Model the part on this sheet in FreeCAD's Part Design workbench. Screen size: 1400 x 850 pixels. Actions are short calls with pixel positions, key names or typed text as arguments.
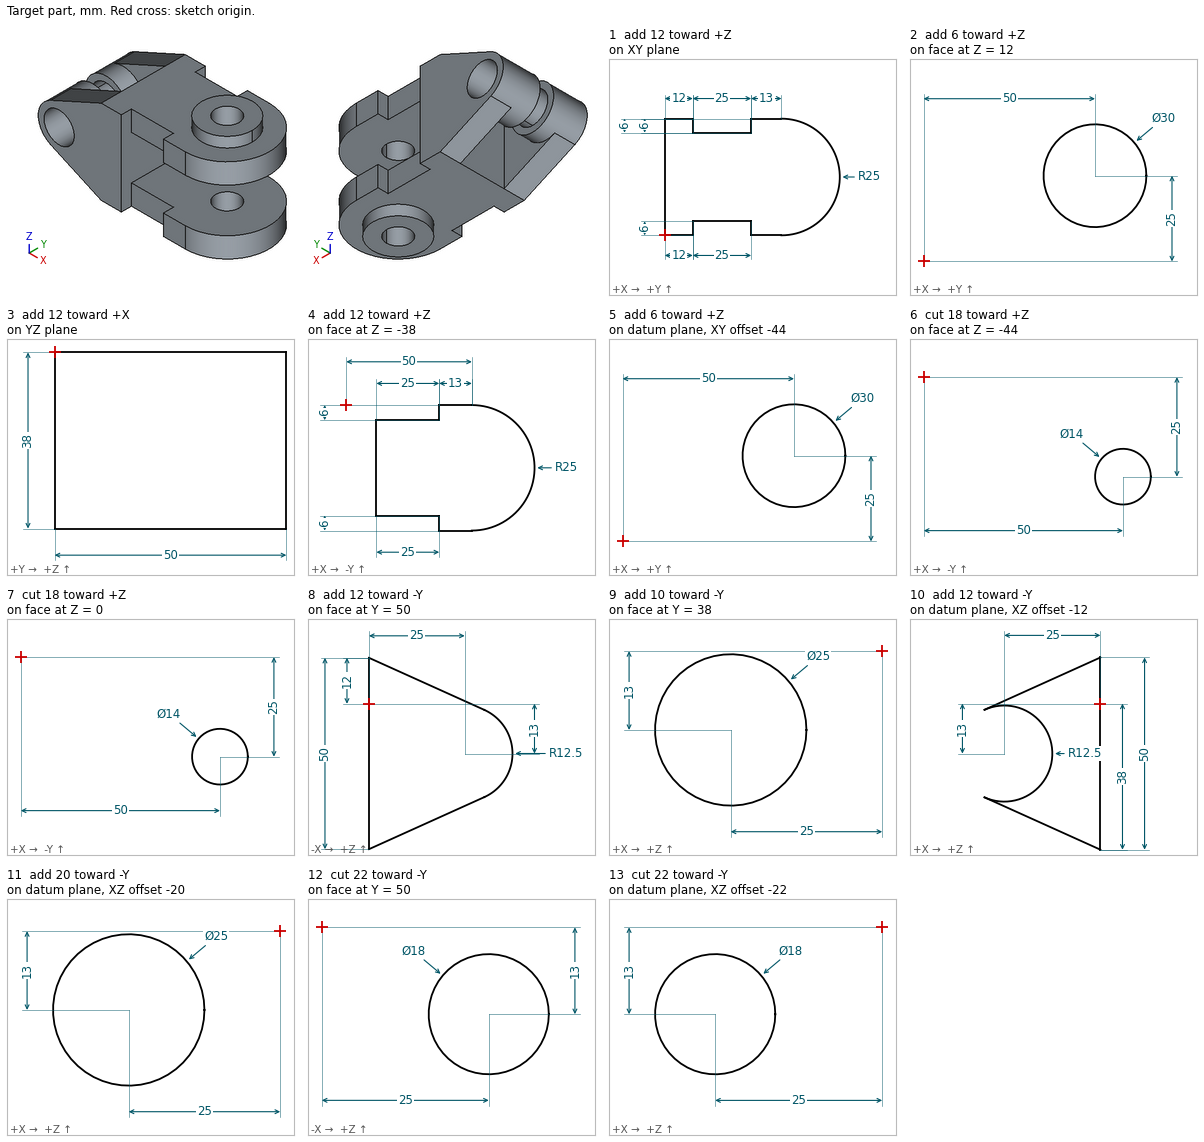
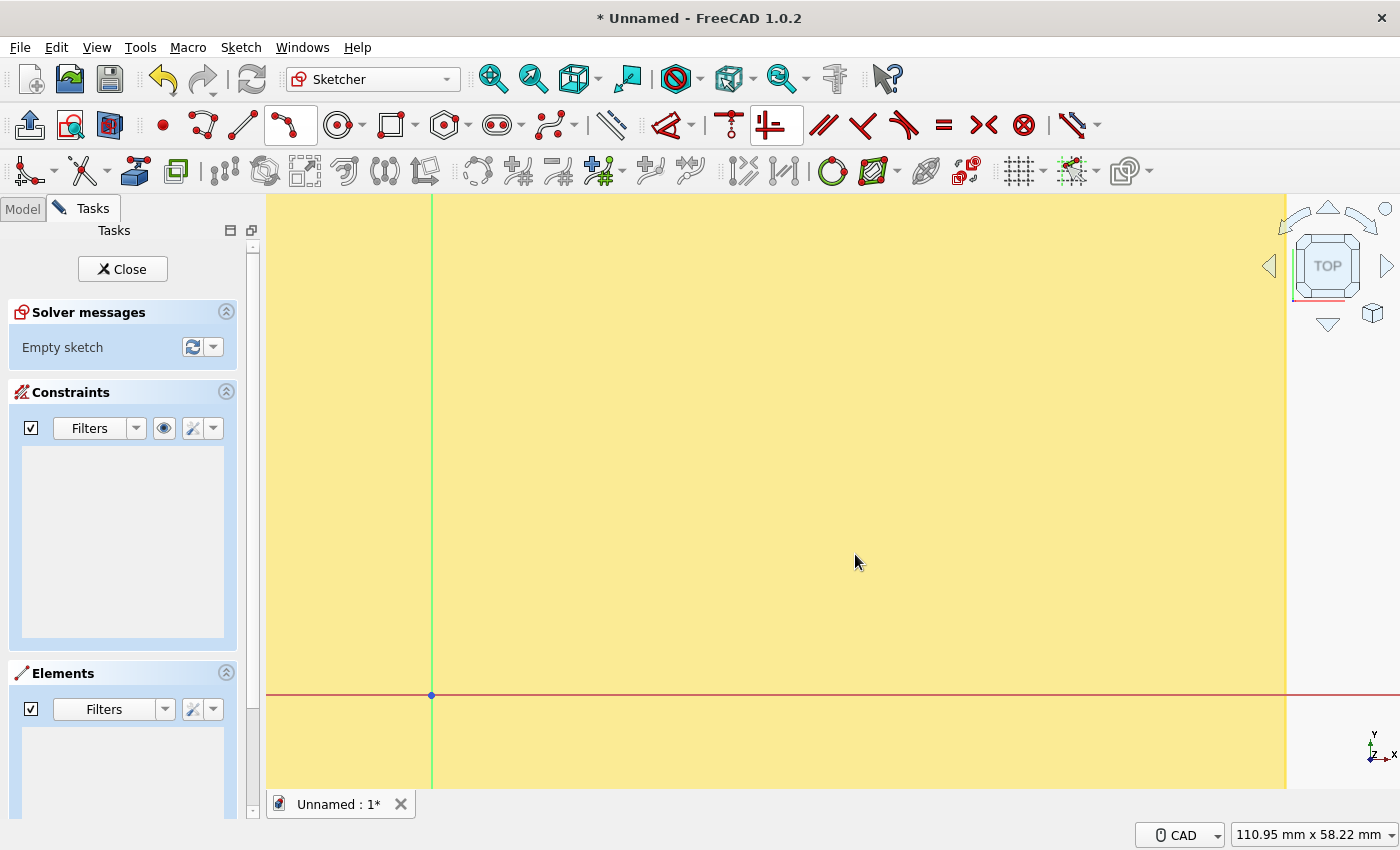
click(338, 126)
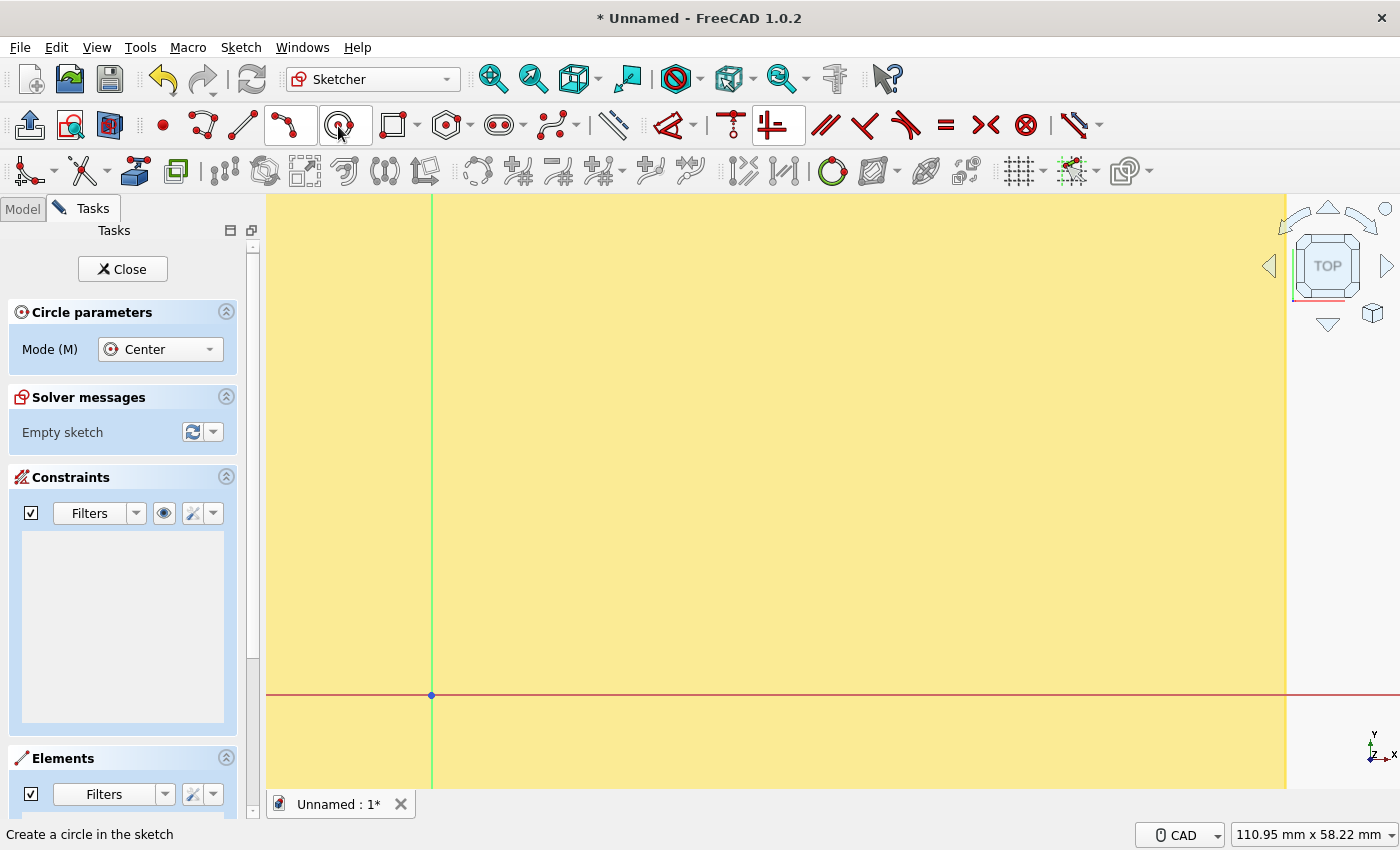
click(943, 440)
click(1051, 331)
key(Escape)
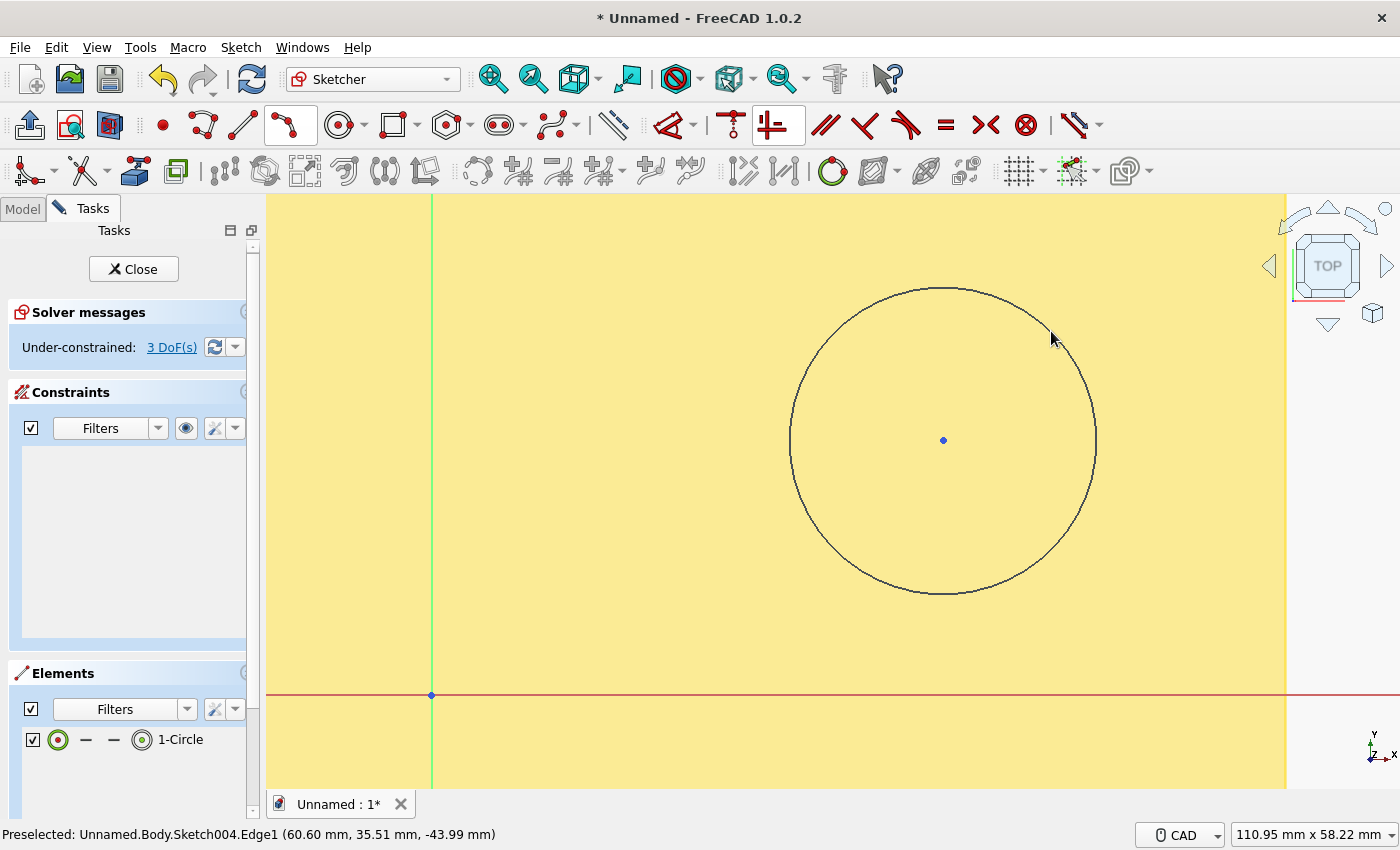
click(668, 126)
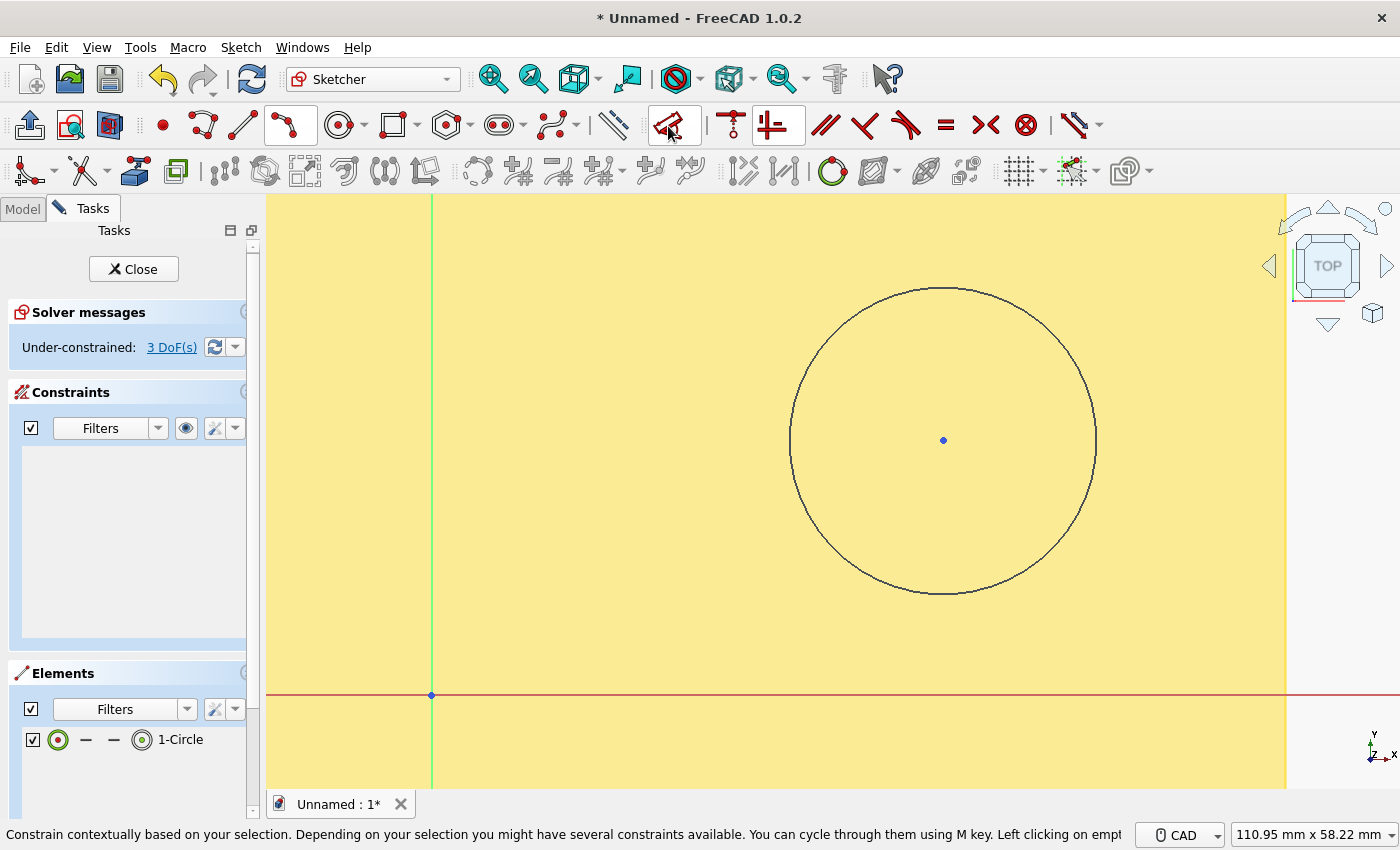
click(1051, 332)
click(1074, 309)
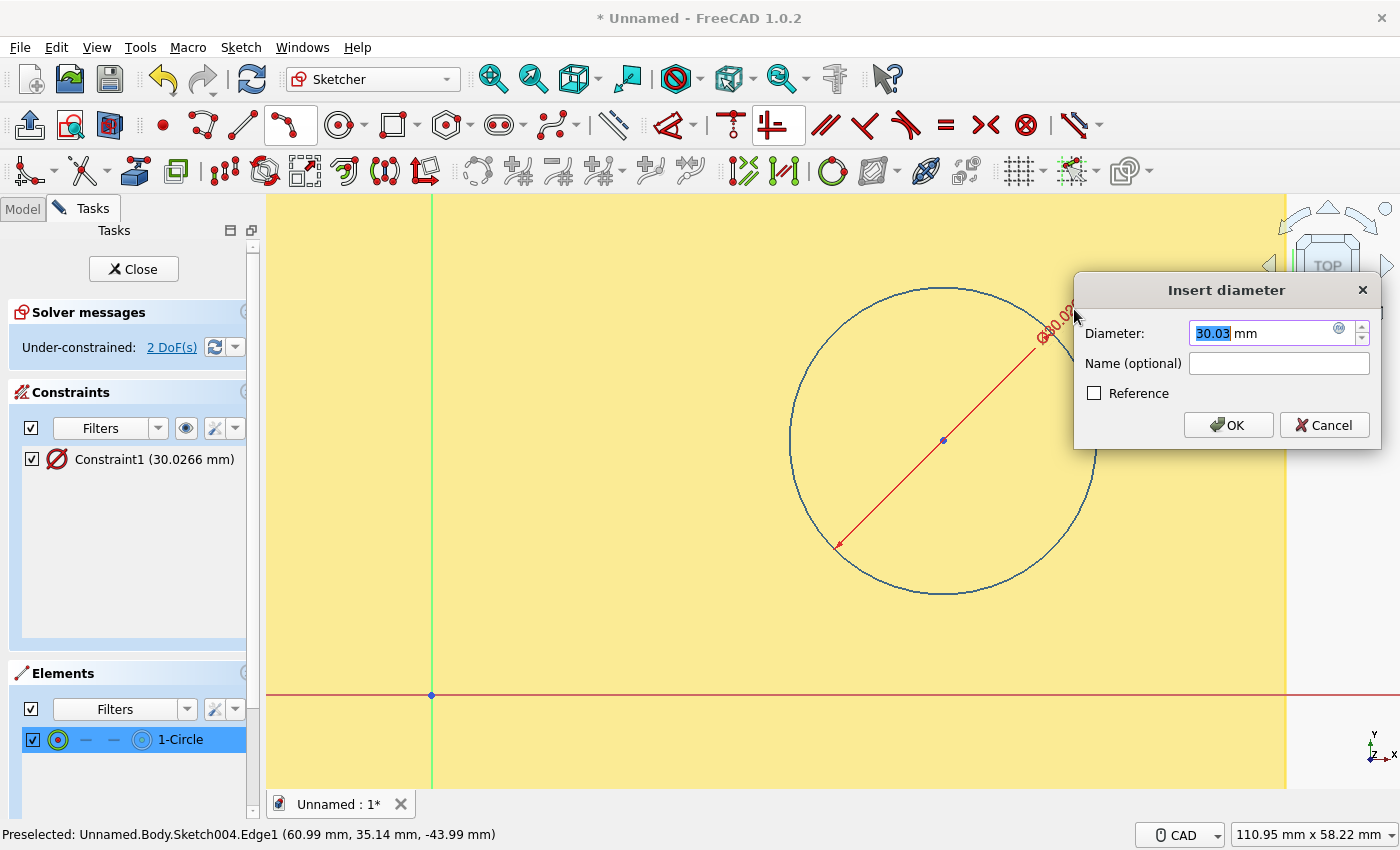
text(30)
key(Return)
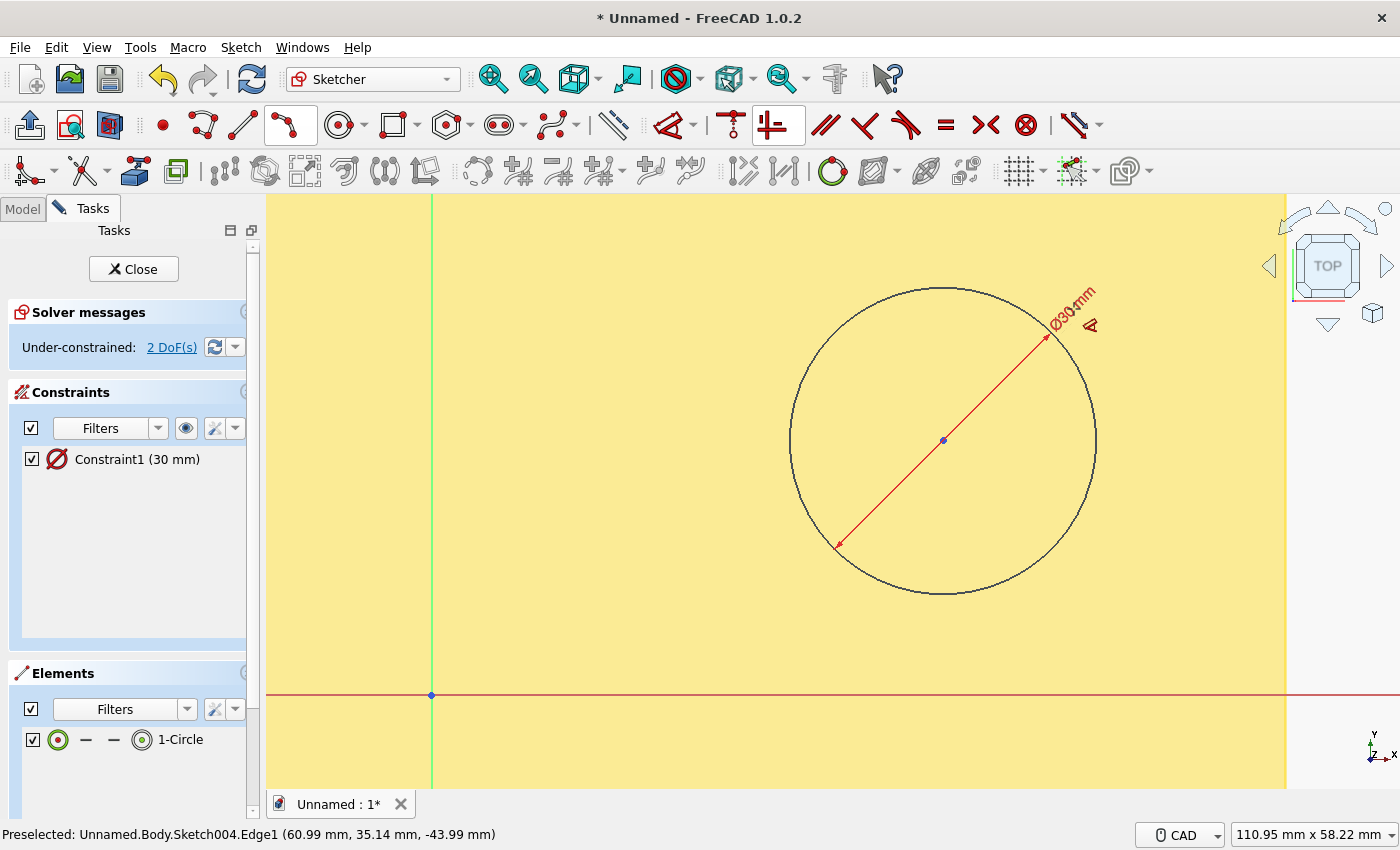
click(943, 441)
click(687, 729)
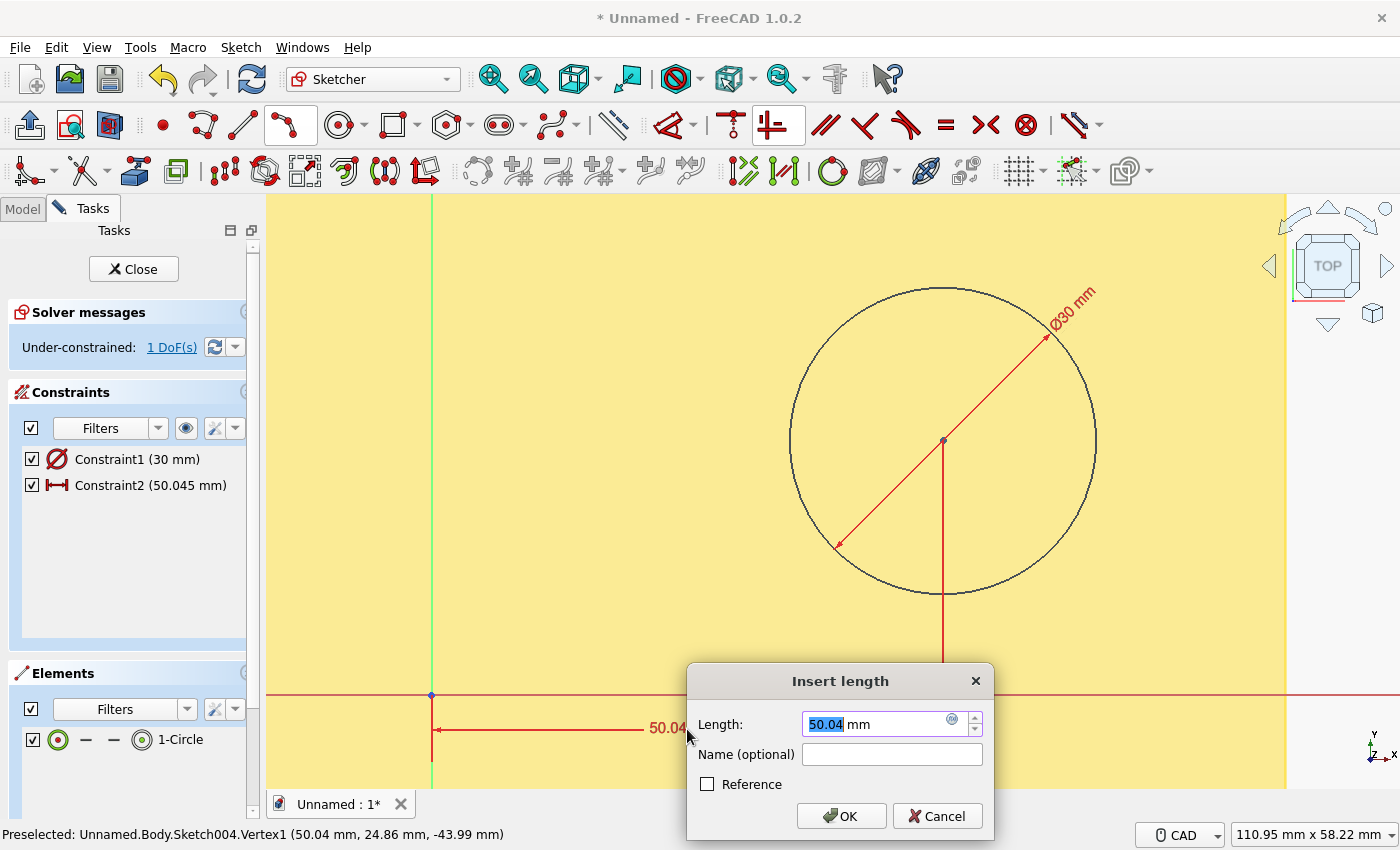
text(50)
key(Return)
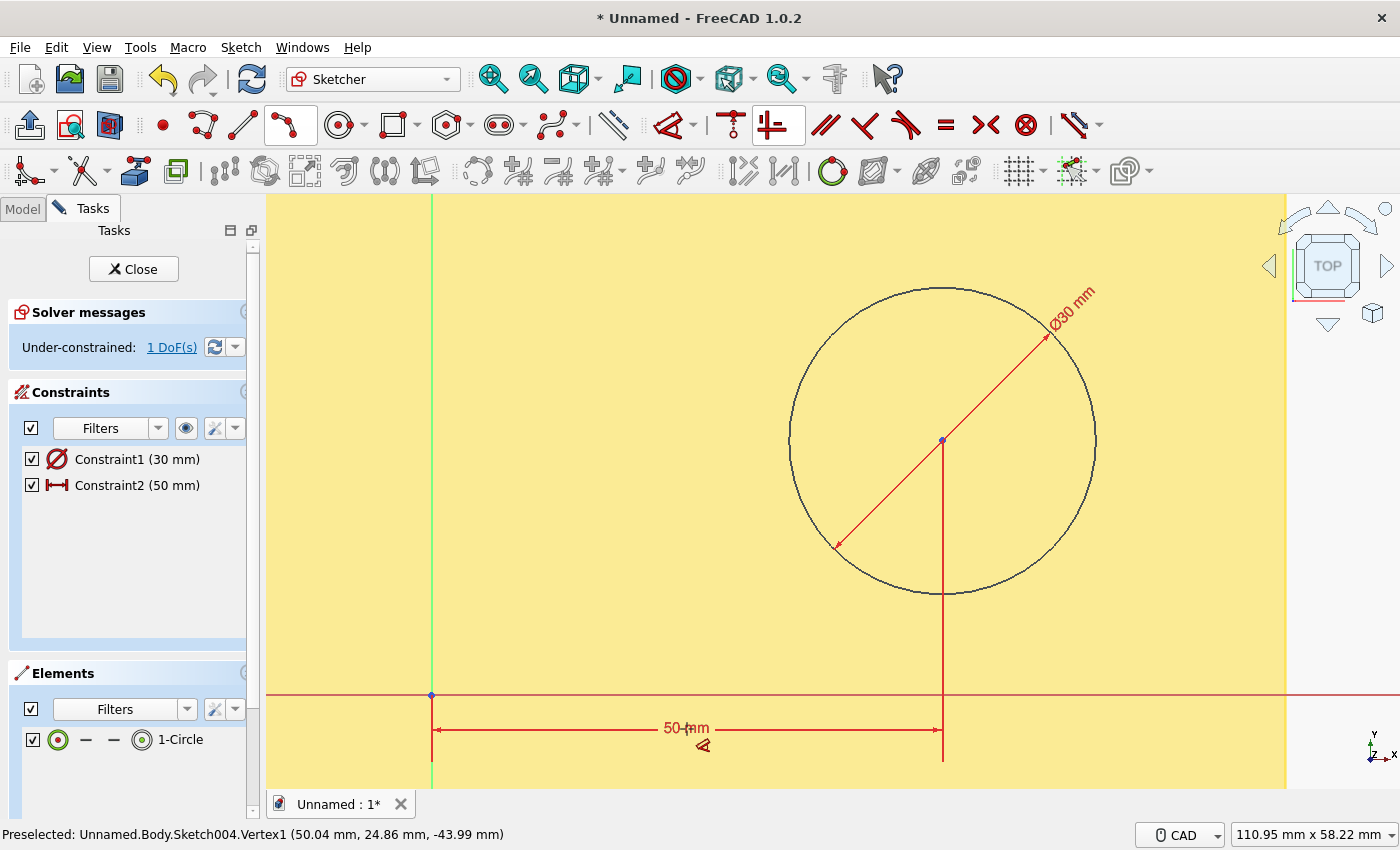
click(943, 441)
click(398, 568)